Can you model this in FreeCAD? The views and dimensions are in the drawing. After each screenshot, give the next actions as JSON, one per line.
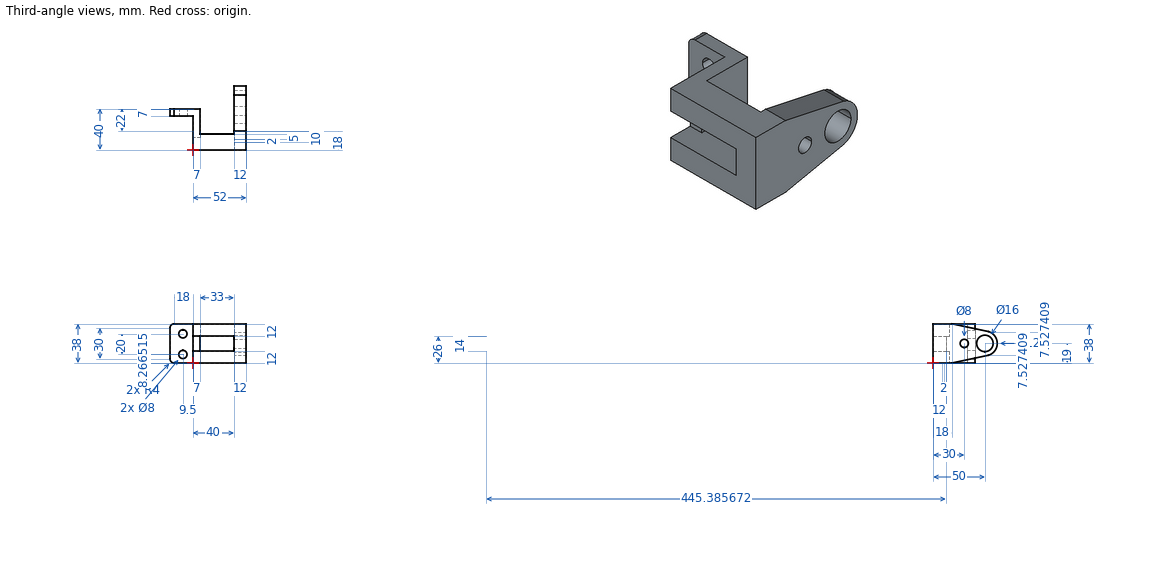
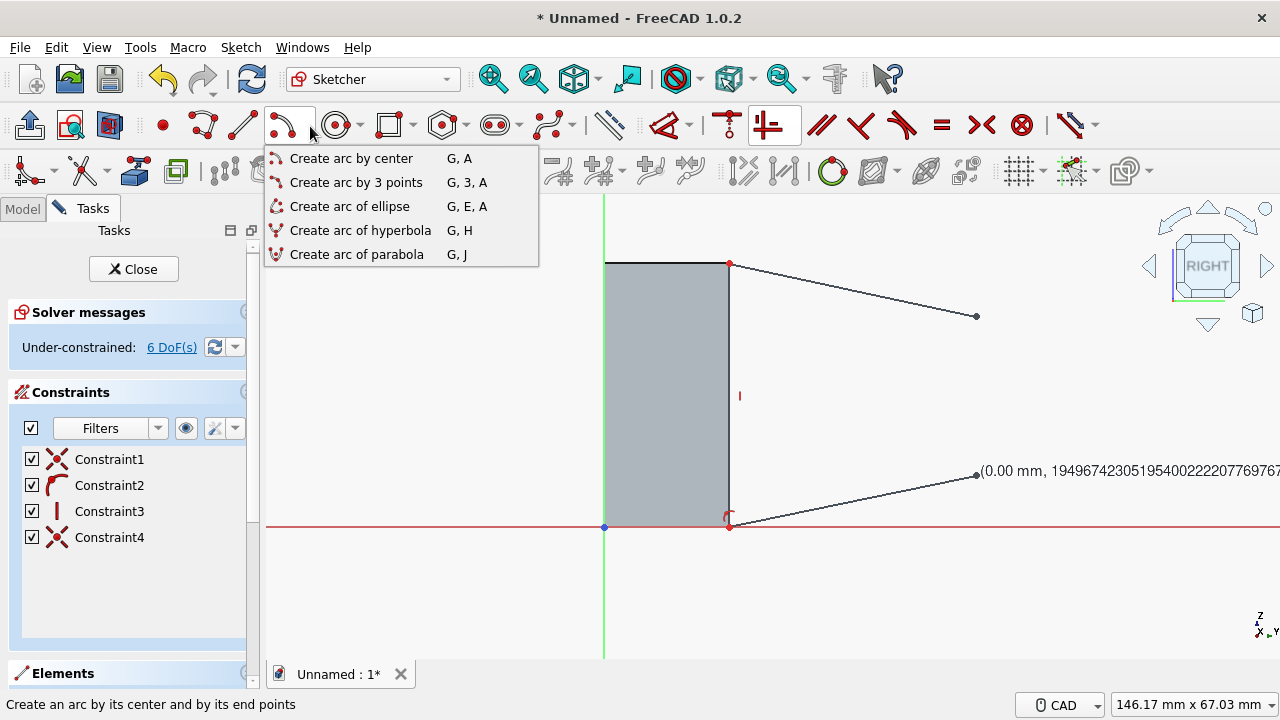
{"action": "left_click", "coordinate": [402, 182]}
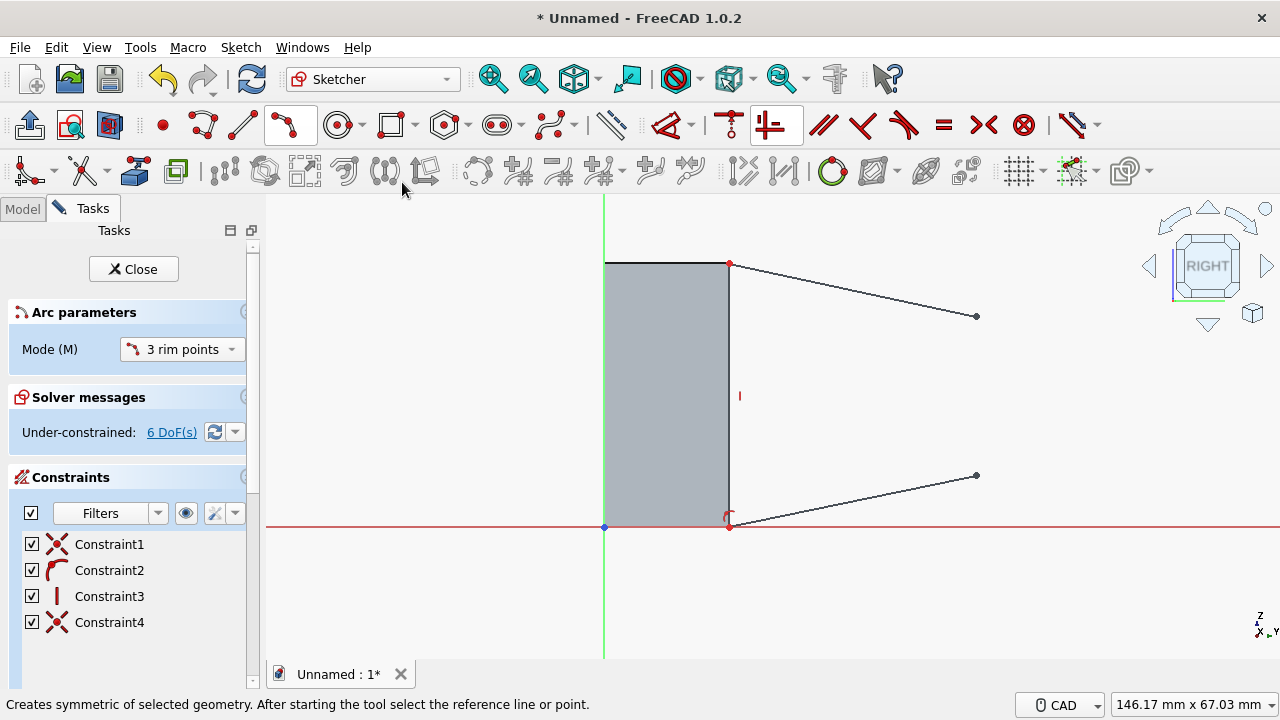
{"action": "left_click", "coordinate": [976, 476]}
{"action": "left_click", "coordinate": [976, 317]}
{"action": "left_click", "coordinate": [1034, 395]}
{"action": "key", "text": "Escape"}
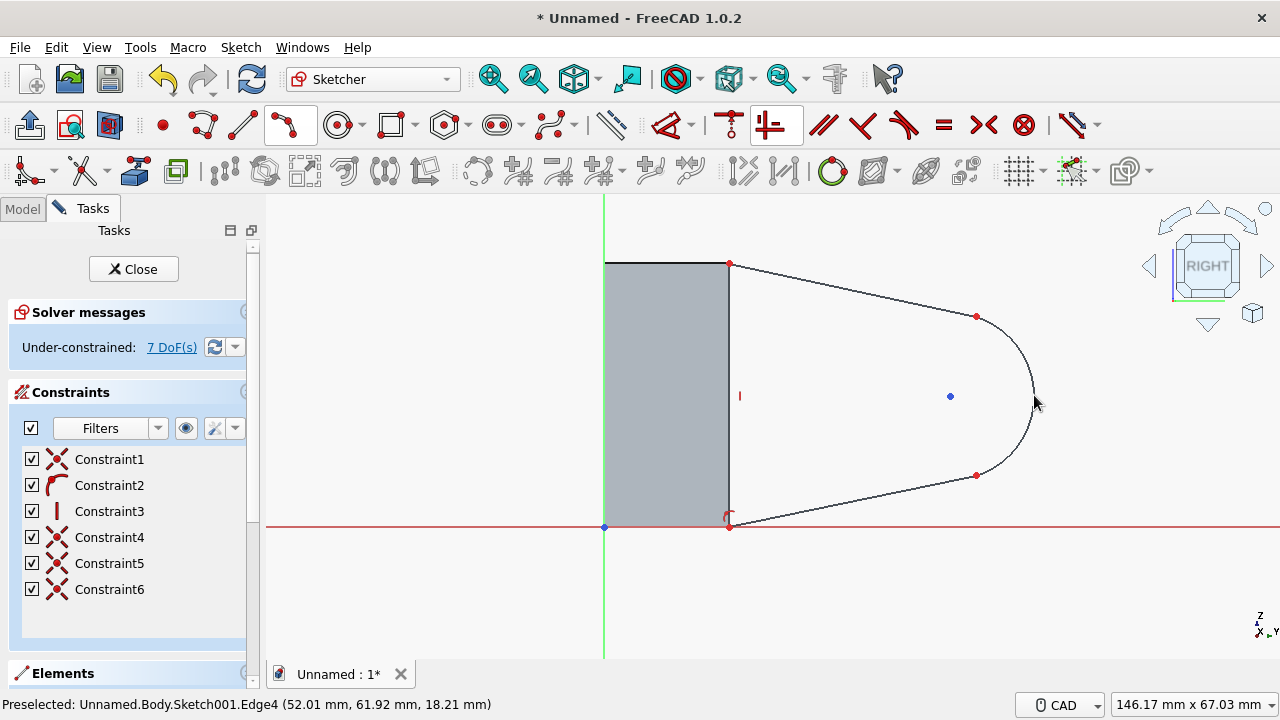
{"action": "left_click", "coordinate": [666, 126]}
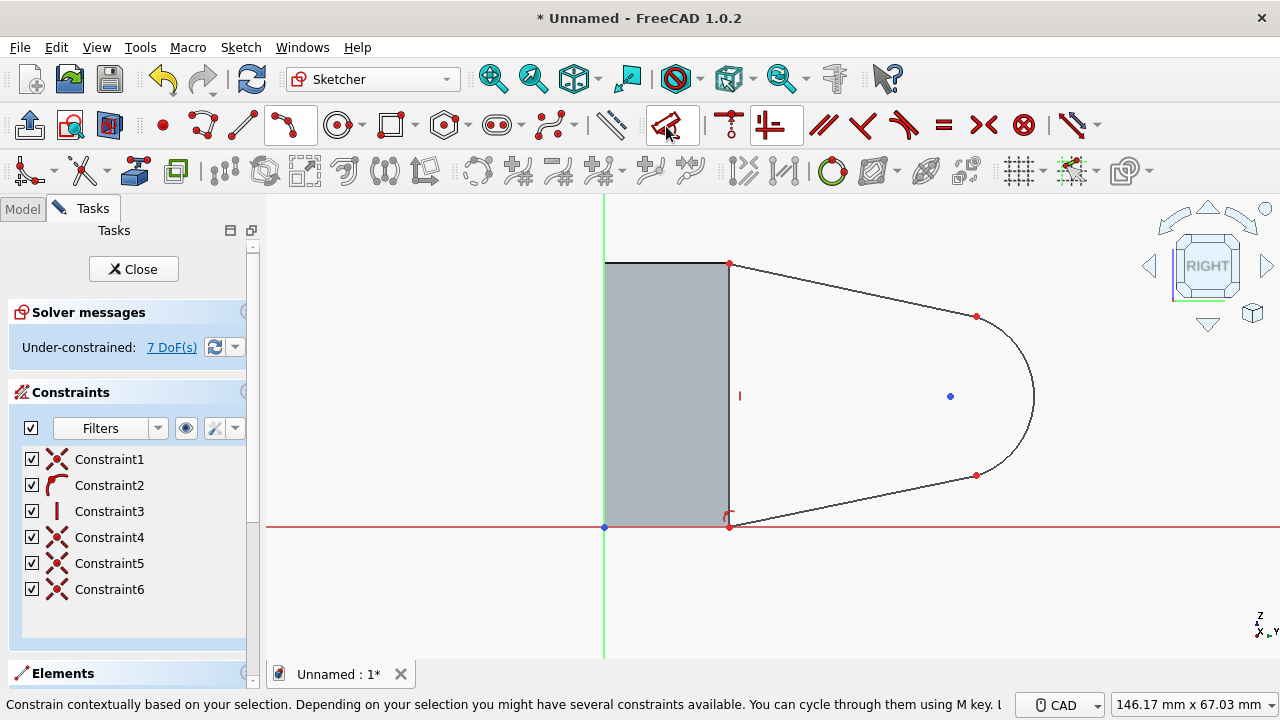
{"action": "left_click", "coordinate": [1024, 437]}
{"action": "left_click", "coordinate": [1052, 452]}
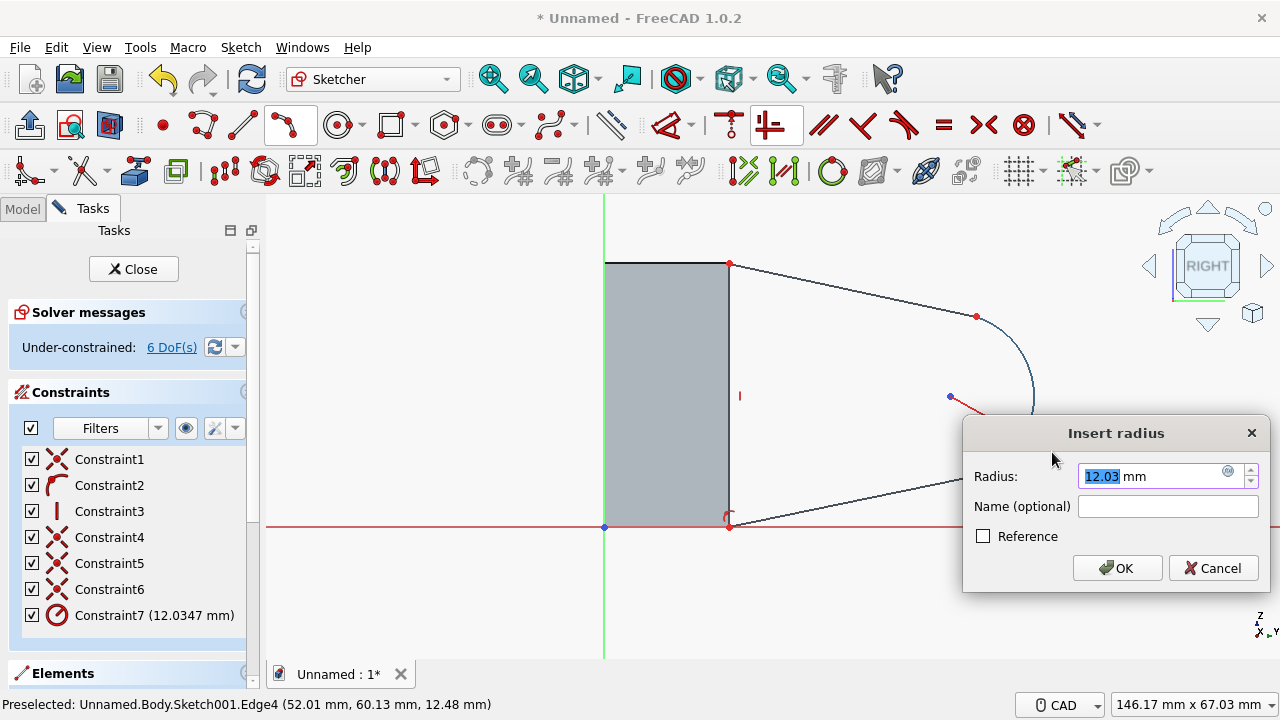
{"action": "type", "text": "12"}
{"action": "key", "text": "Return"}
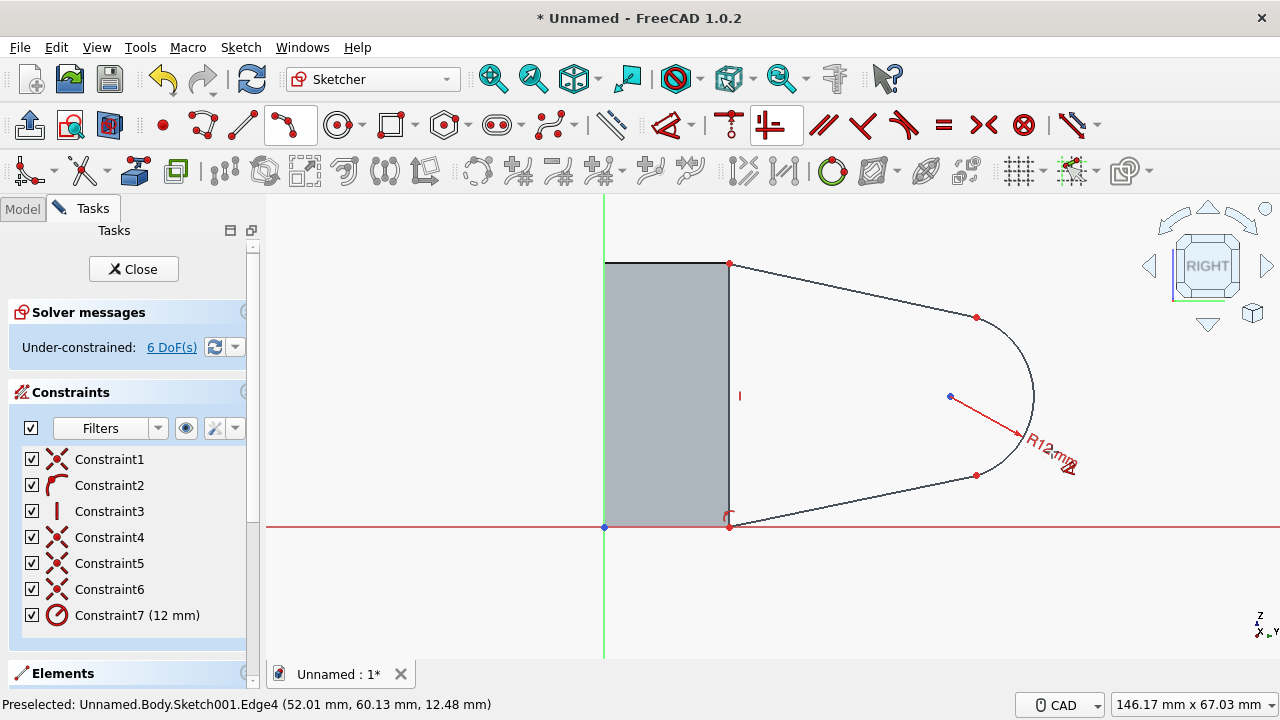
{"action": "left_click", "coordinate": [729, 343]}
{"action": "left_click", "coordinate": [695, 396]}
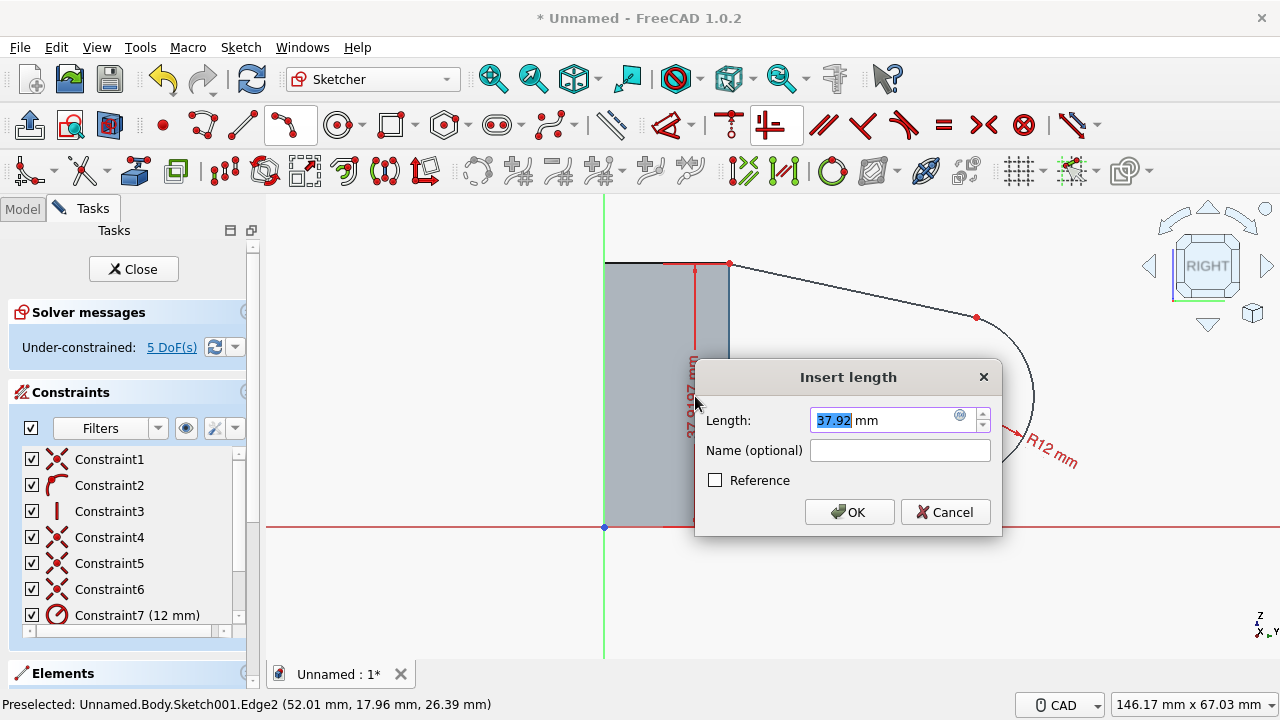
{"action": "type", "text": "38"}
{"action": "key", "text": "Return"}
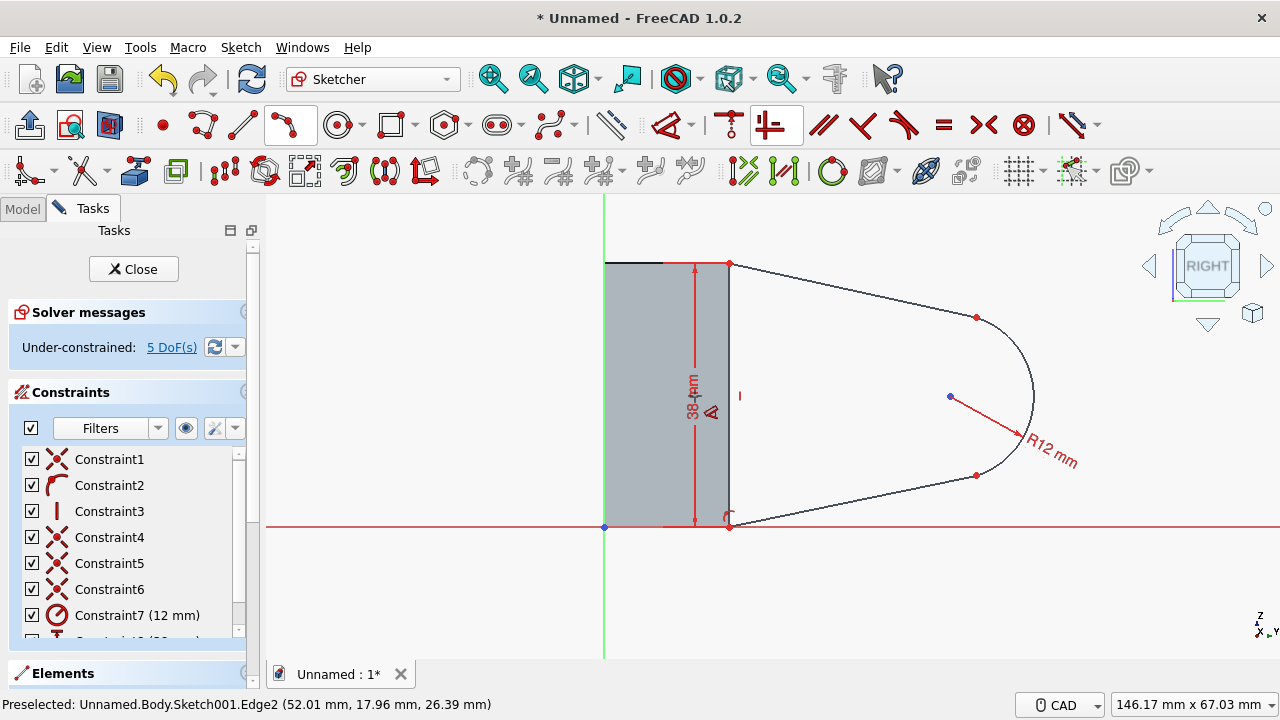
{"action": "left_click", "coordinate": [729, 263]}
{"action": "left_click", "coordinate": [667, 561]}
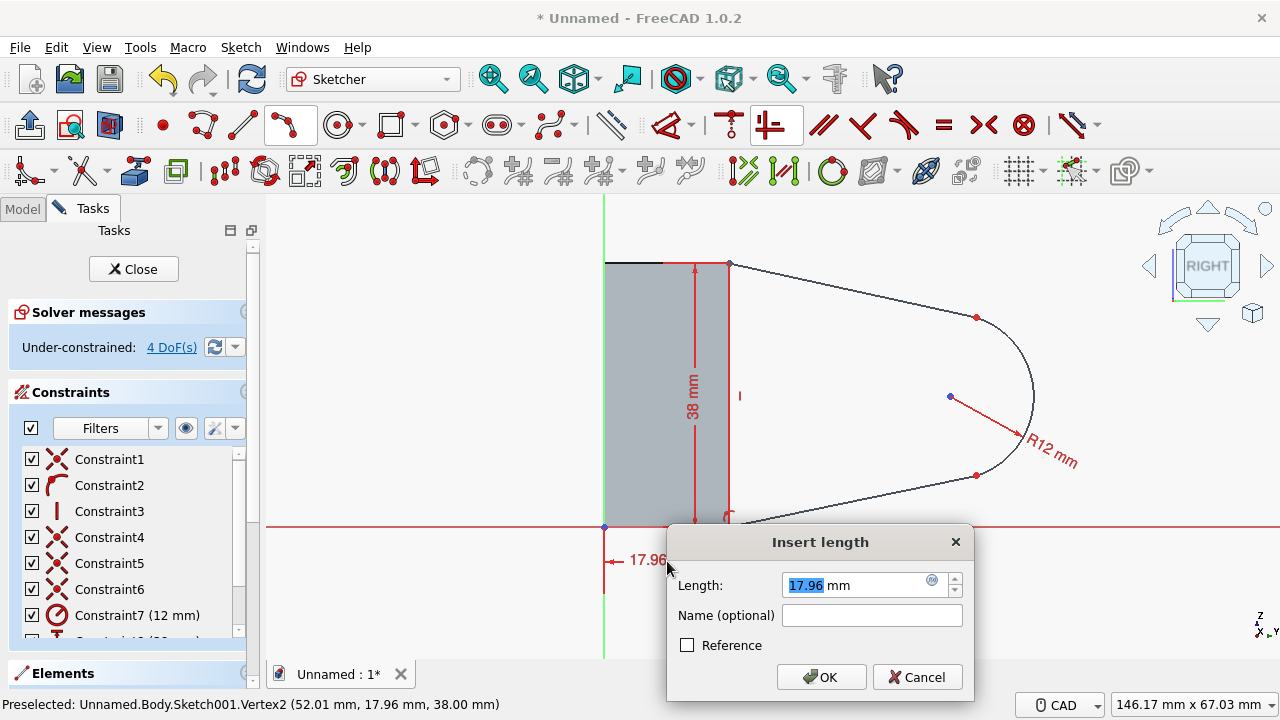
{"action": "type", "text": "18"}
{"action": "key", "text": "Return"}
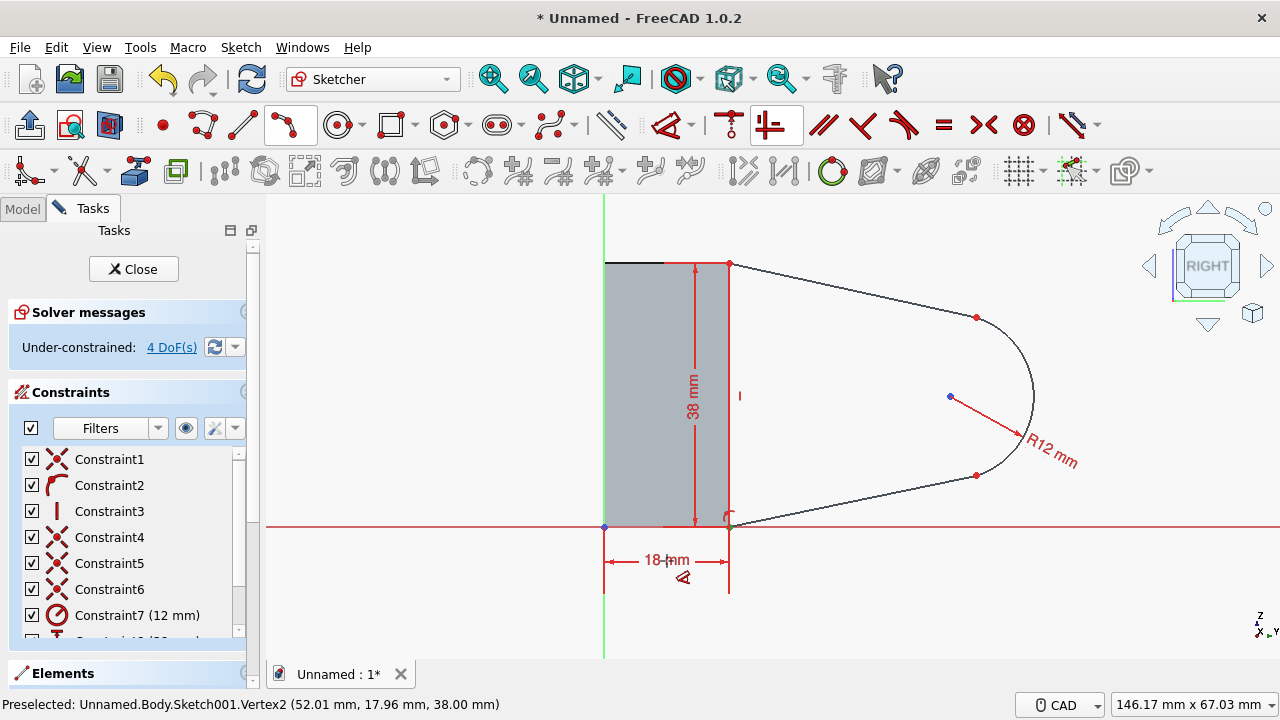
{"action": "left_click", "coordinate": [951, 397]}
{"action": "left_click", "coordinate": [777, 561]}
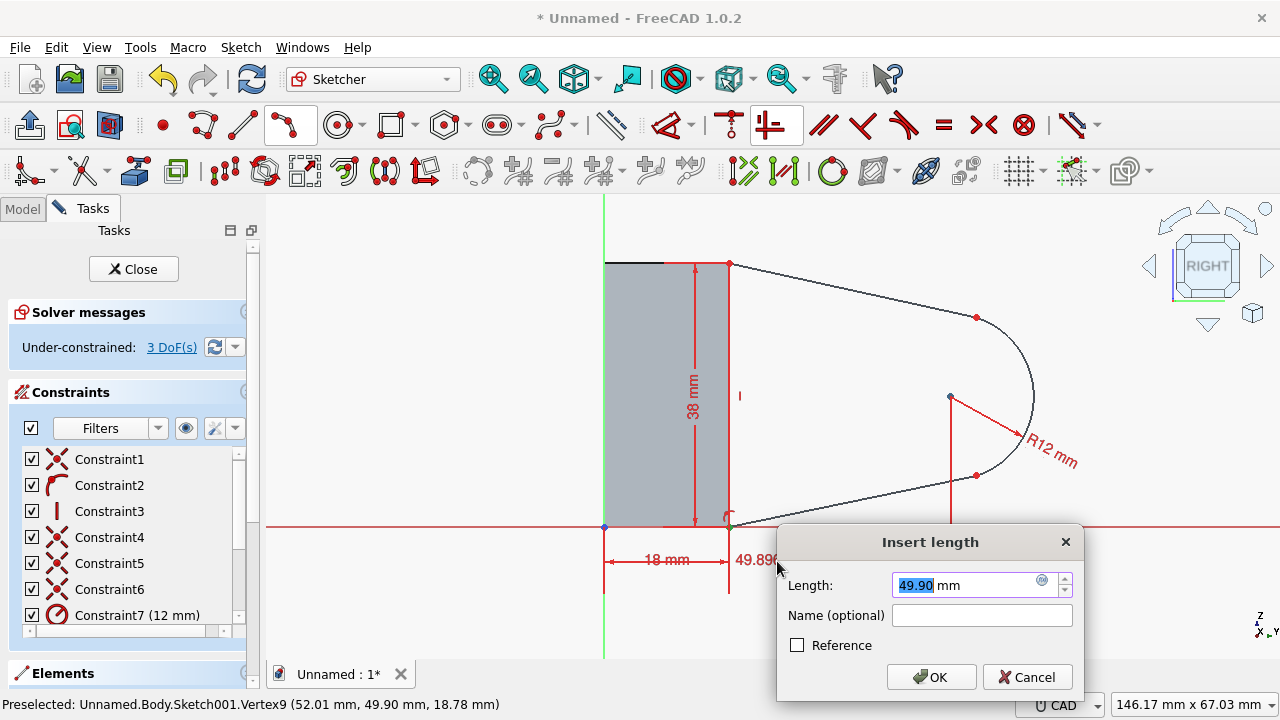
{"action": "type", "text": "50"}
{"action": "key", "text": "Return"}